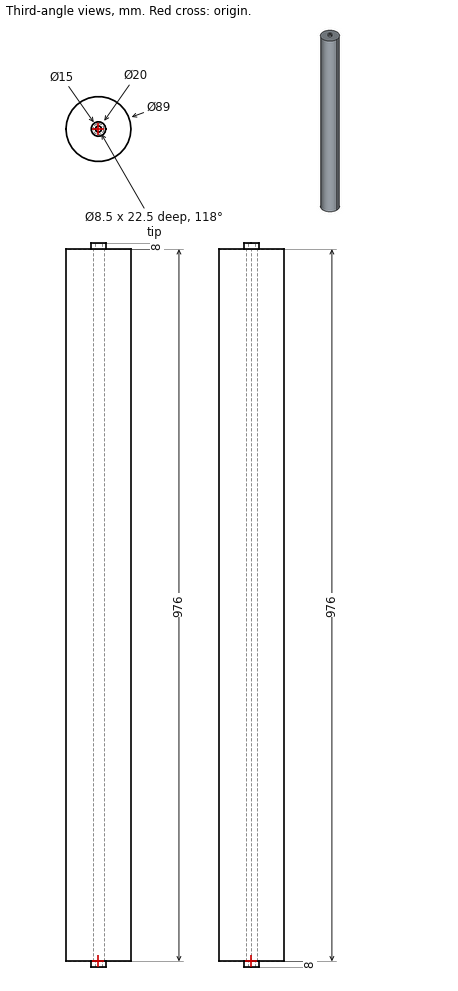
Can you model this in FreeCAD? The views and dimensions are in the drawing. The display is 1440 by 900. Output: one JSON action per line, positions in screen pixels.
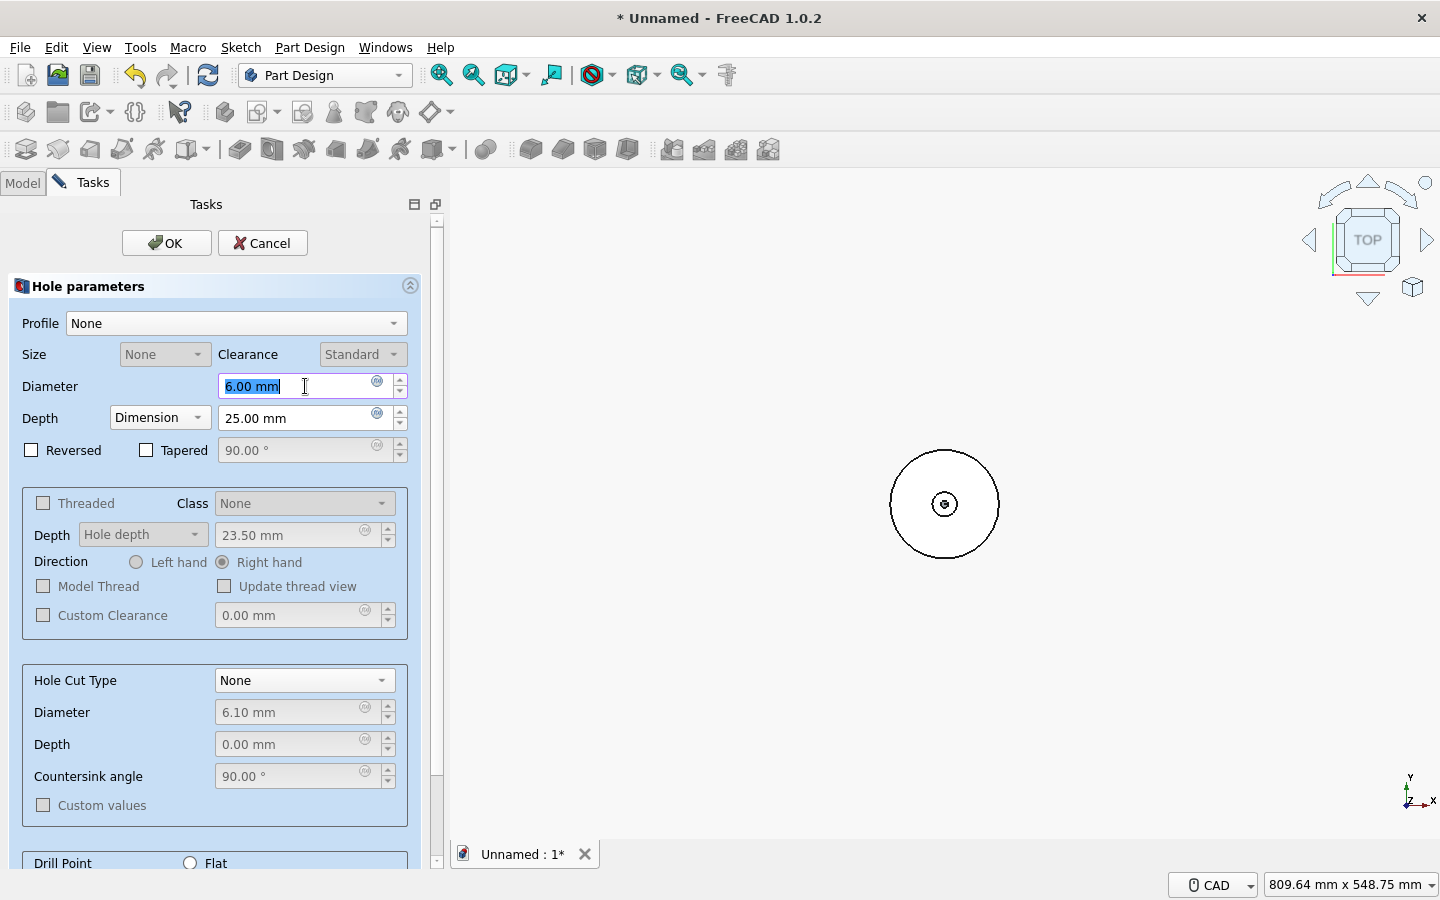
{"action": "type", "text": "8.5"}
{"action": "key", "text": "Tab"}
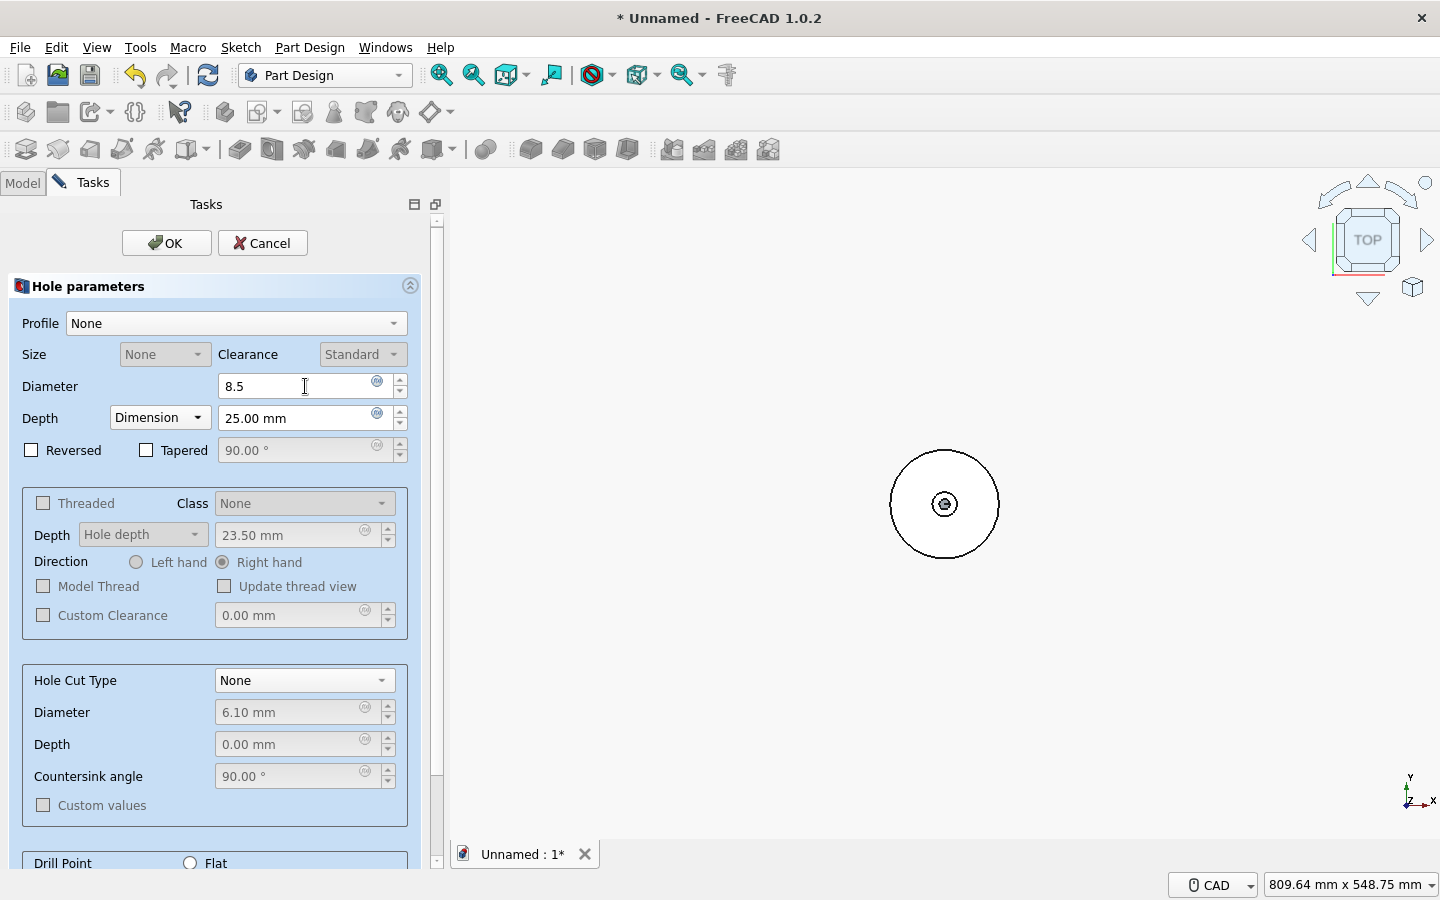
{"action": "triple_click", "coordinate": [305, 418]}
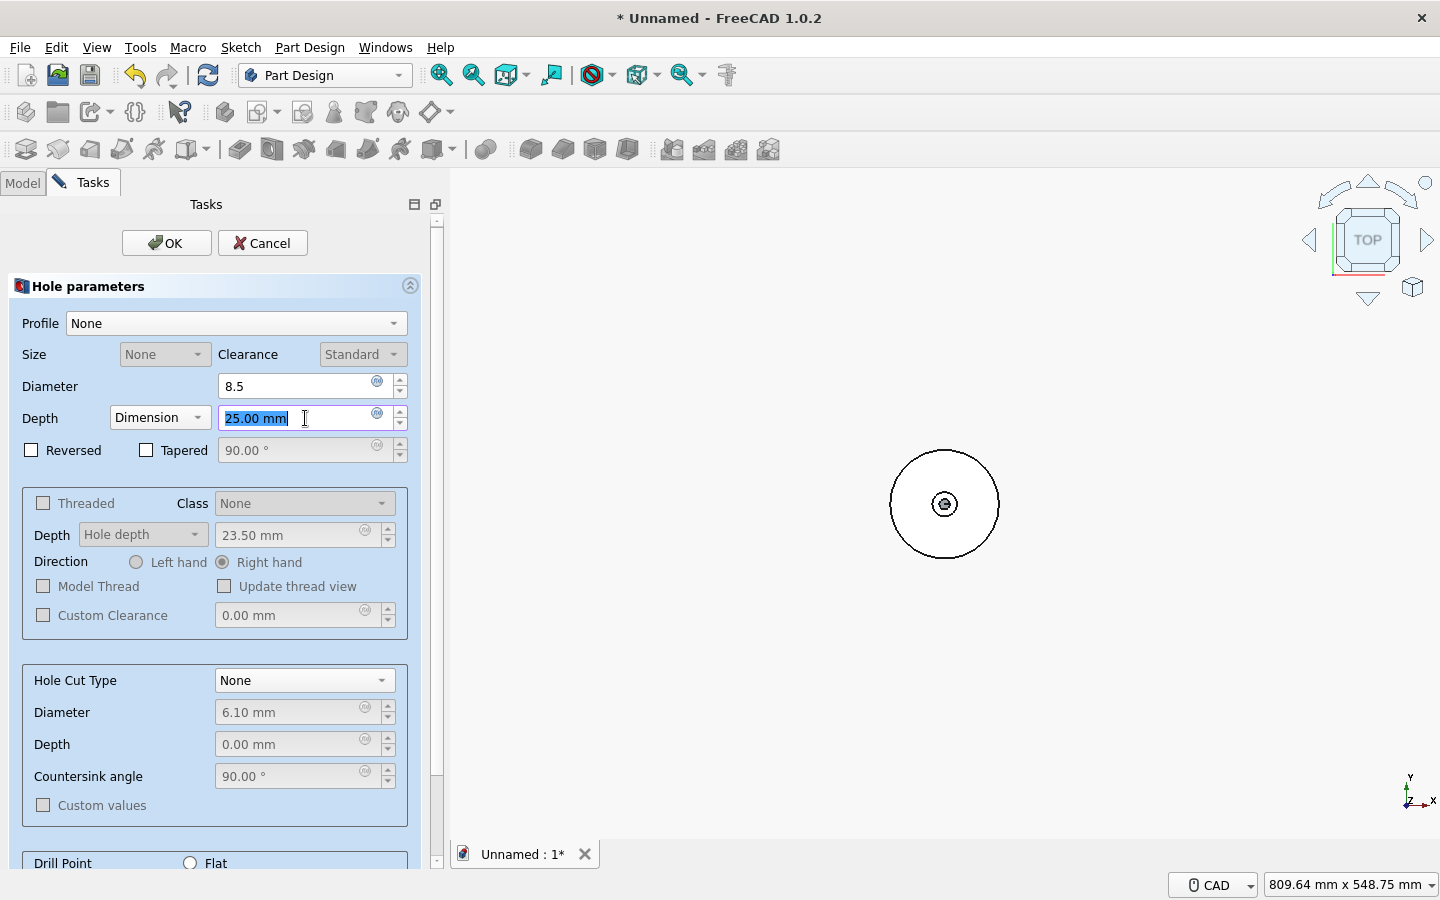
{"action": "type", "text": "22.5"}
{"action": "key", "text": "Tab"}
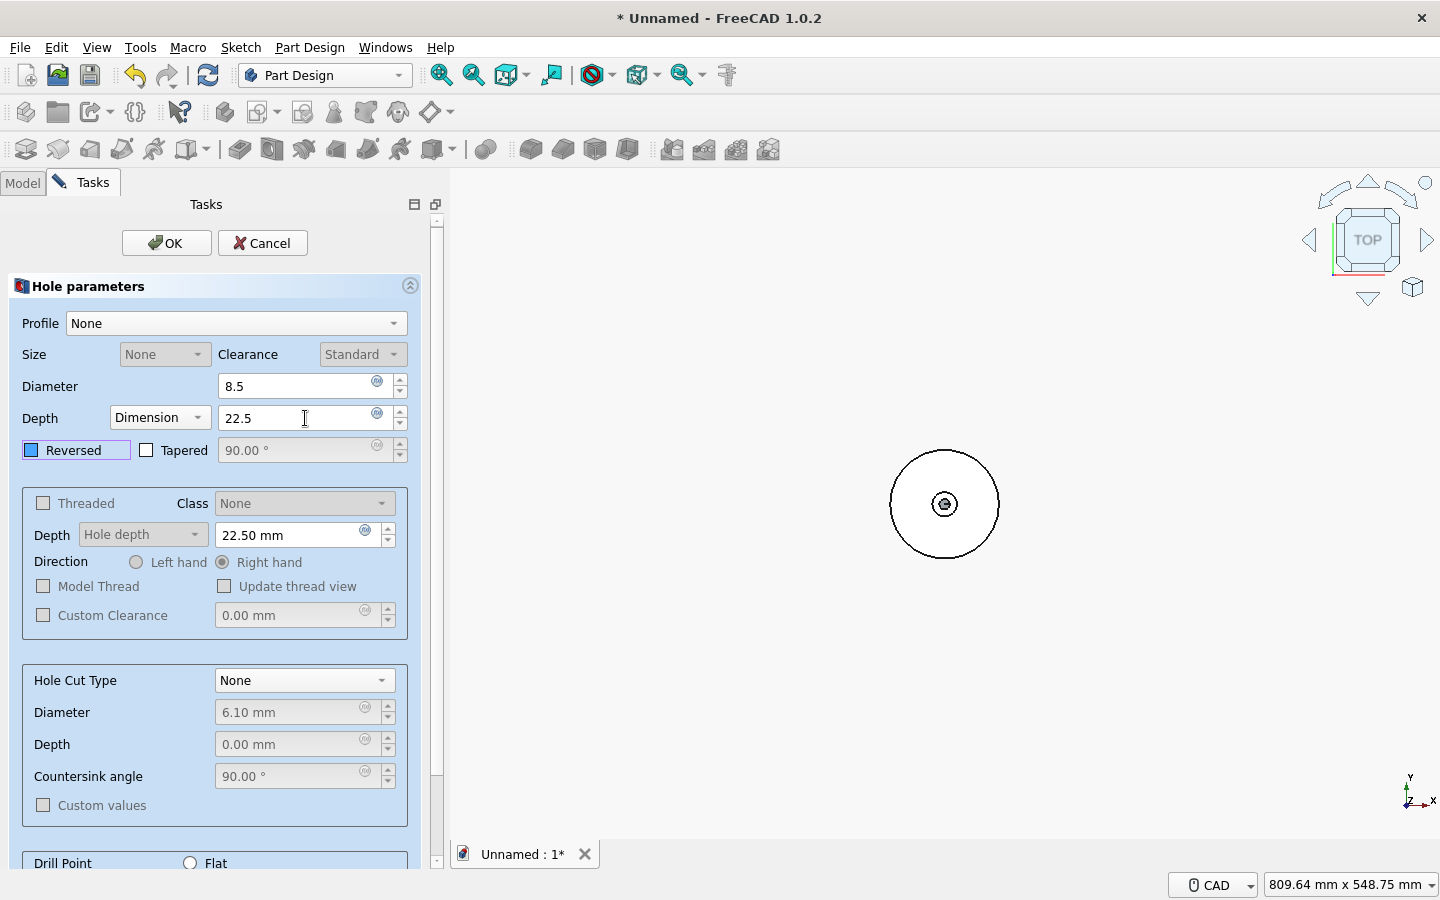
{"action": "left_click", "coordinate": [167, 243]}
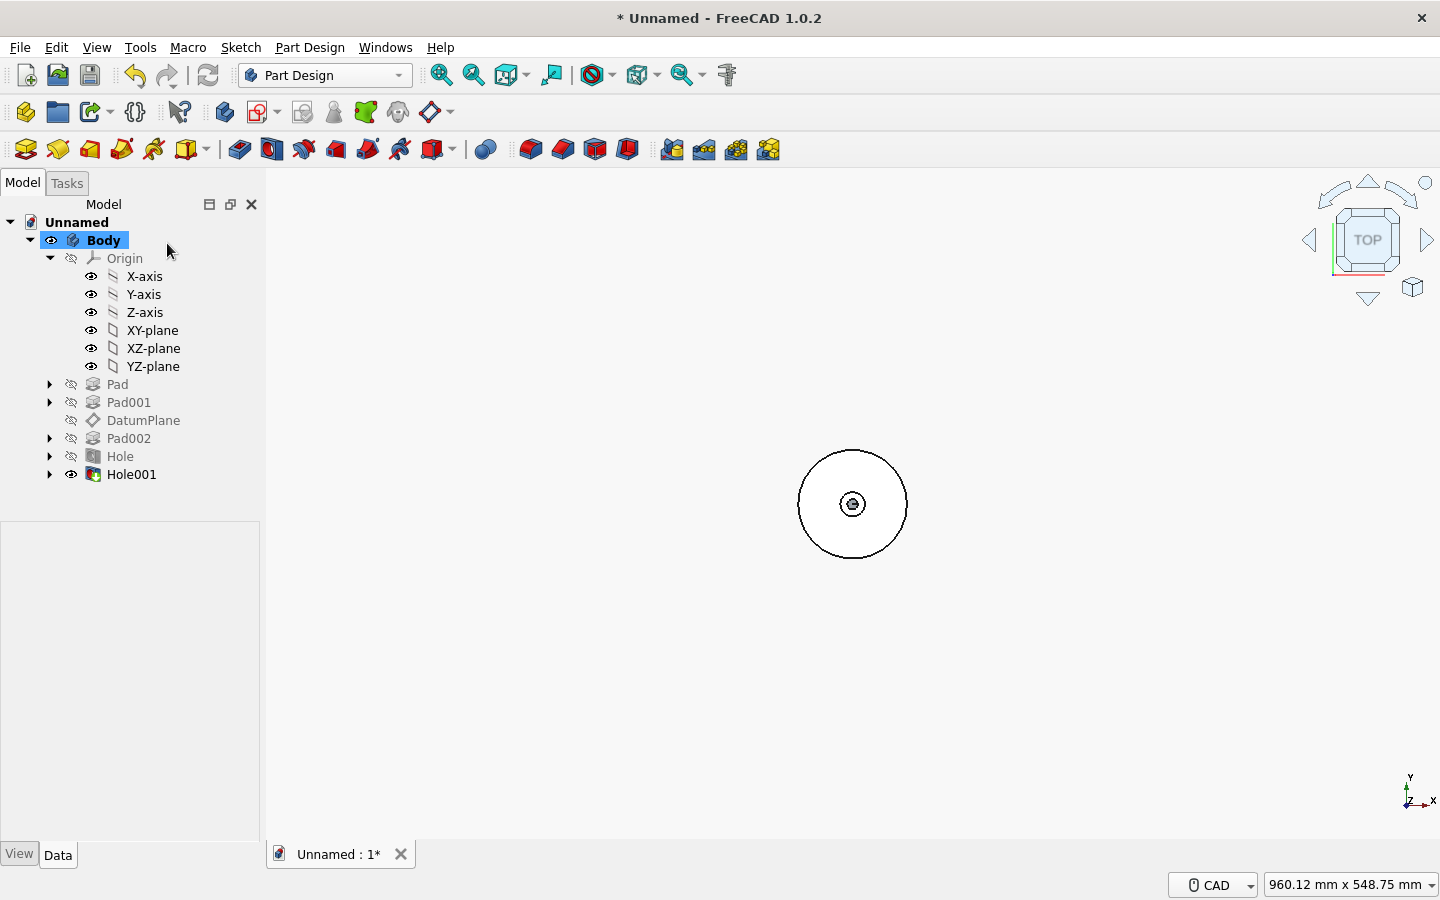
{"action": "left_click", "coordinate": [442, 76]}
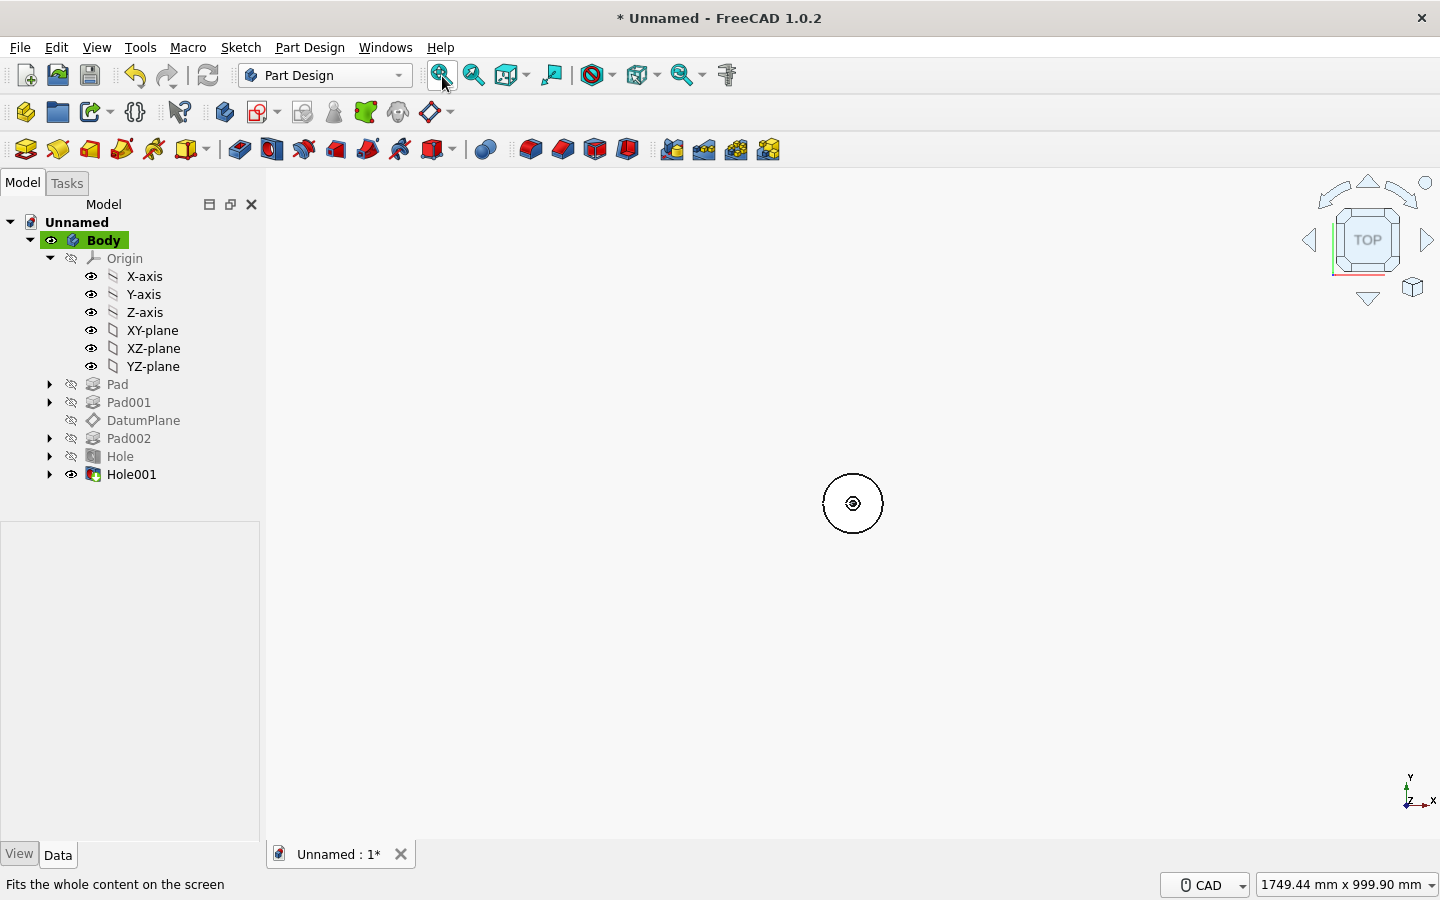
{"action": "left_click", "coordinate": [136, 330]}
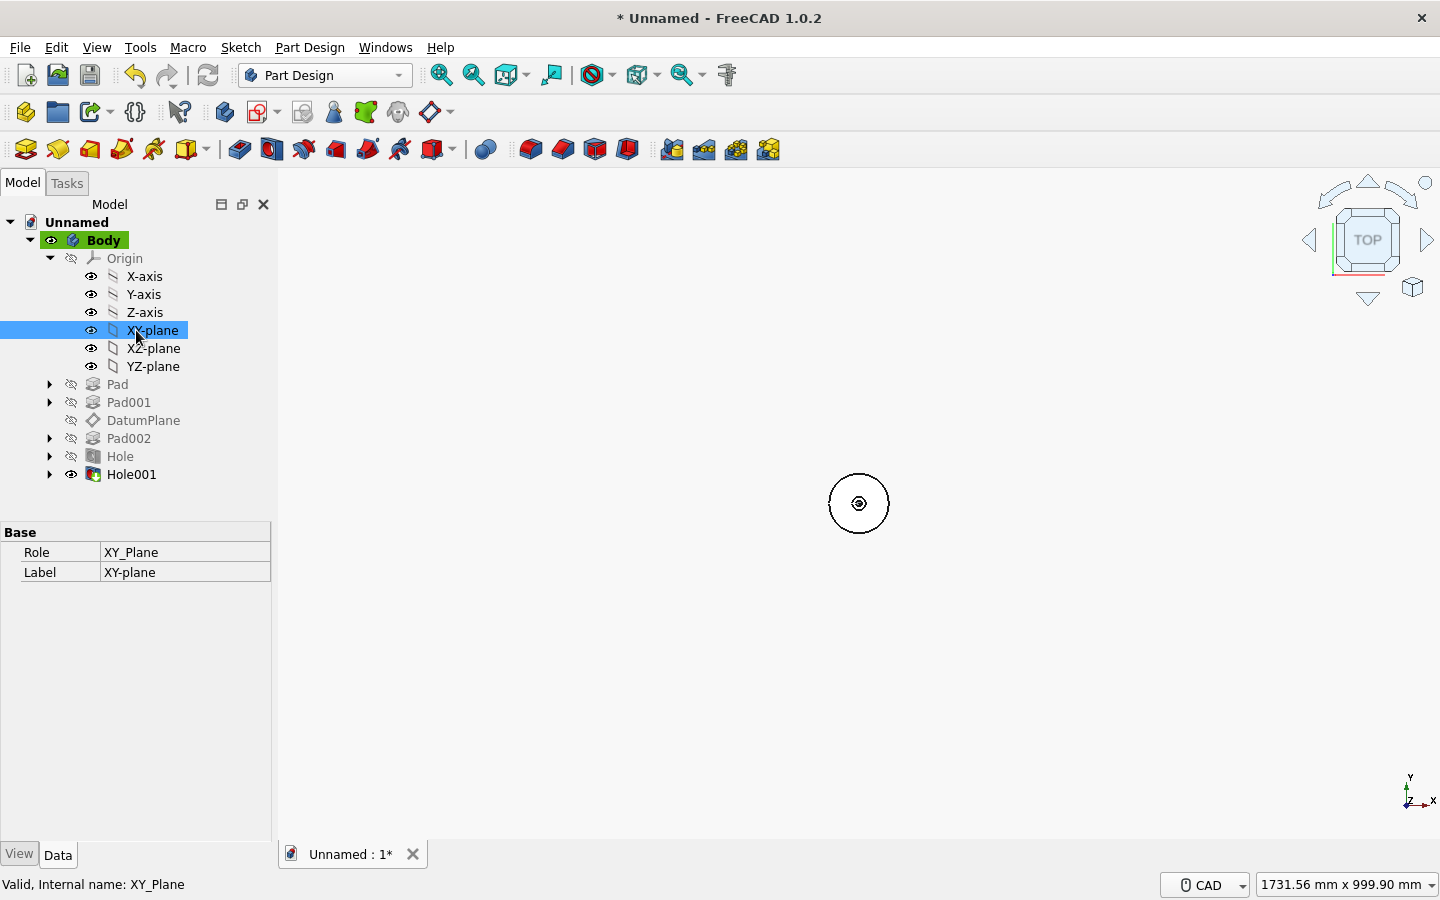
{"action": "left_click", "coordinate": [430, 112]}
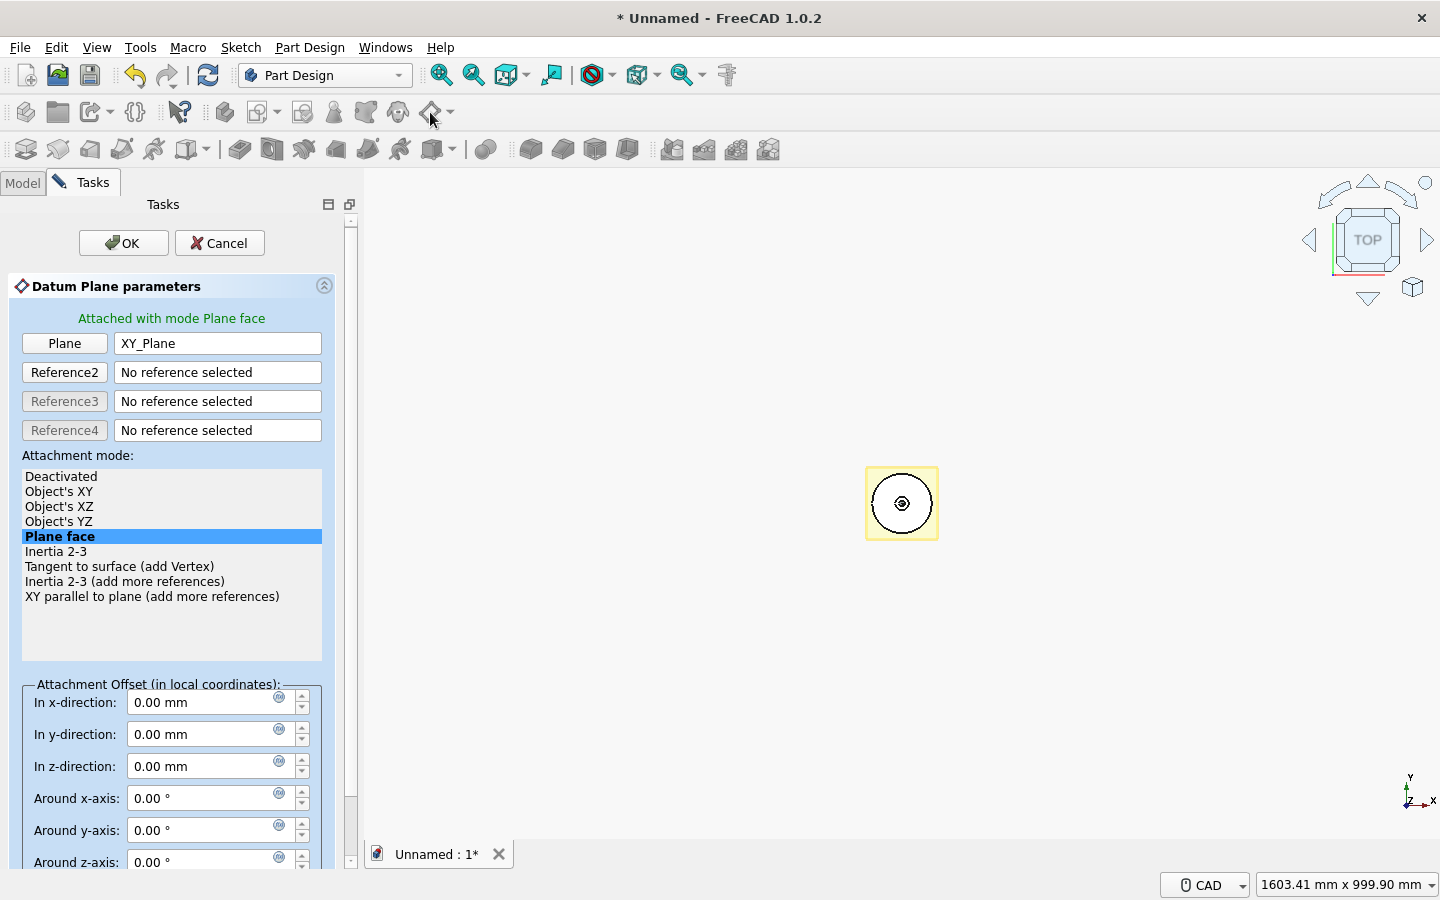
{"action": "triple_click", "coordinate": [210, 766]}